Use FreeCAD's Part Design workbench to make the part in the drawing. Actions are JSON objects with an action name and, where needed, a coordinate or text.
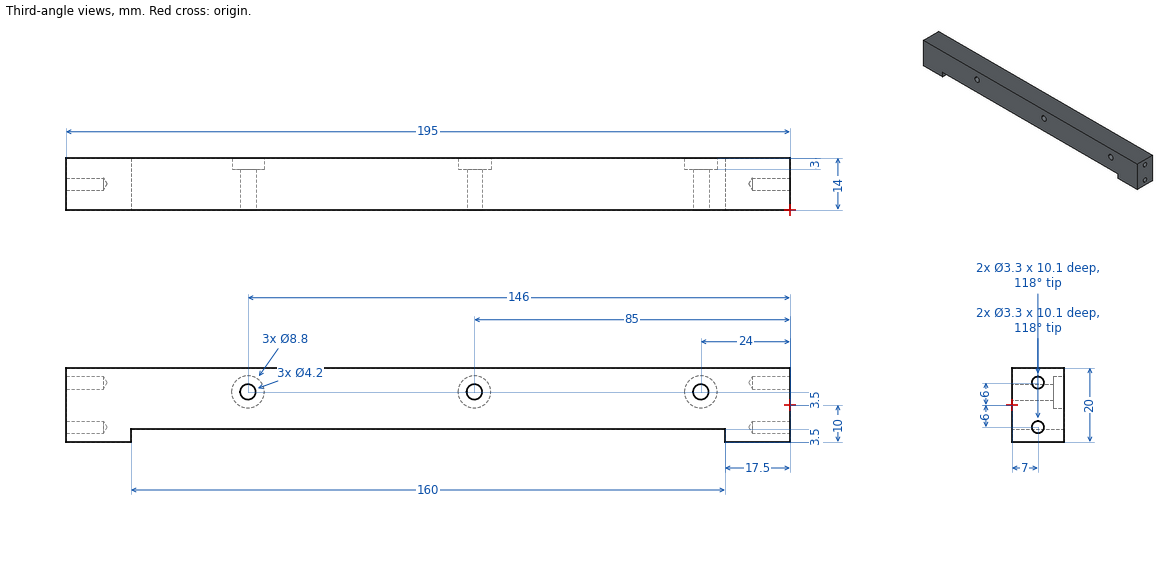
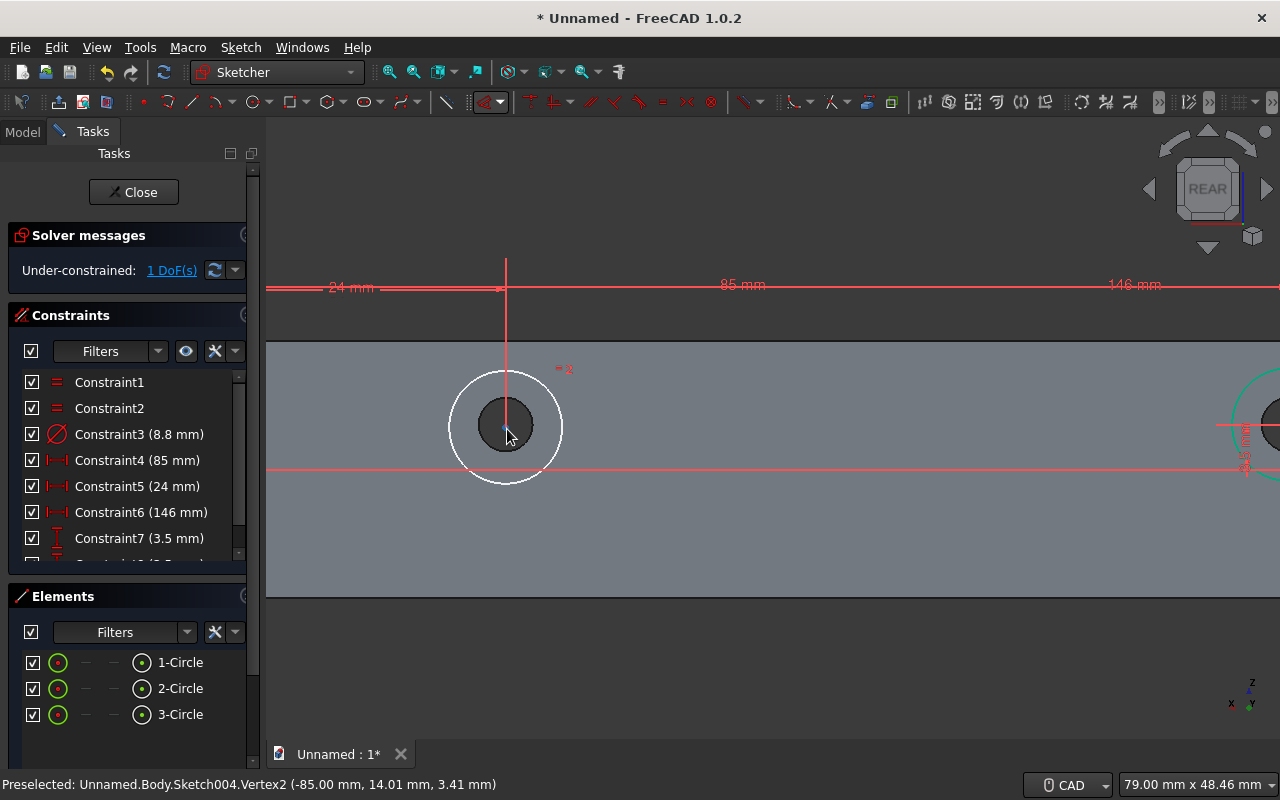
{"action": "left_click", "coordinate": [506, 427]}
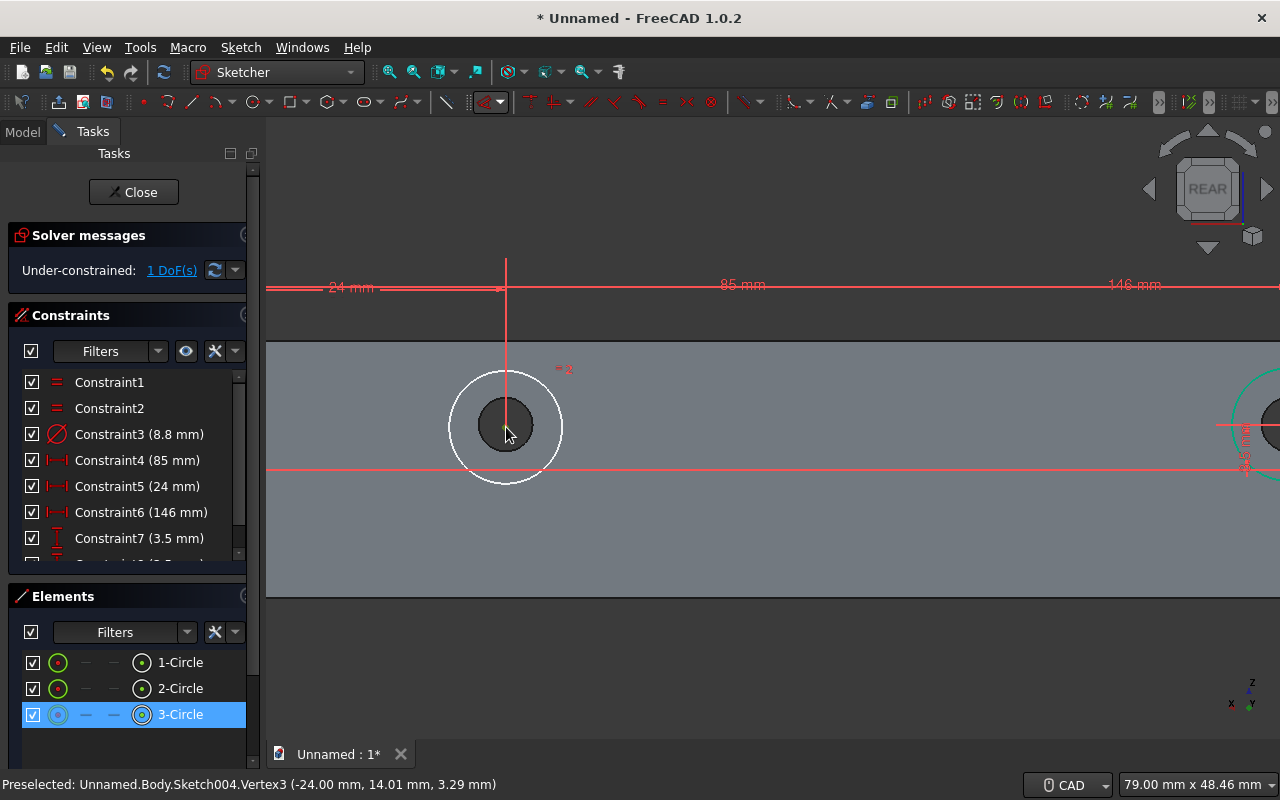
{"action": "key", "text": "i"}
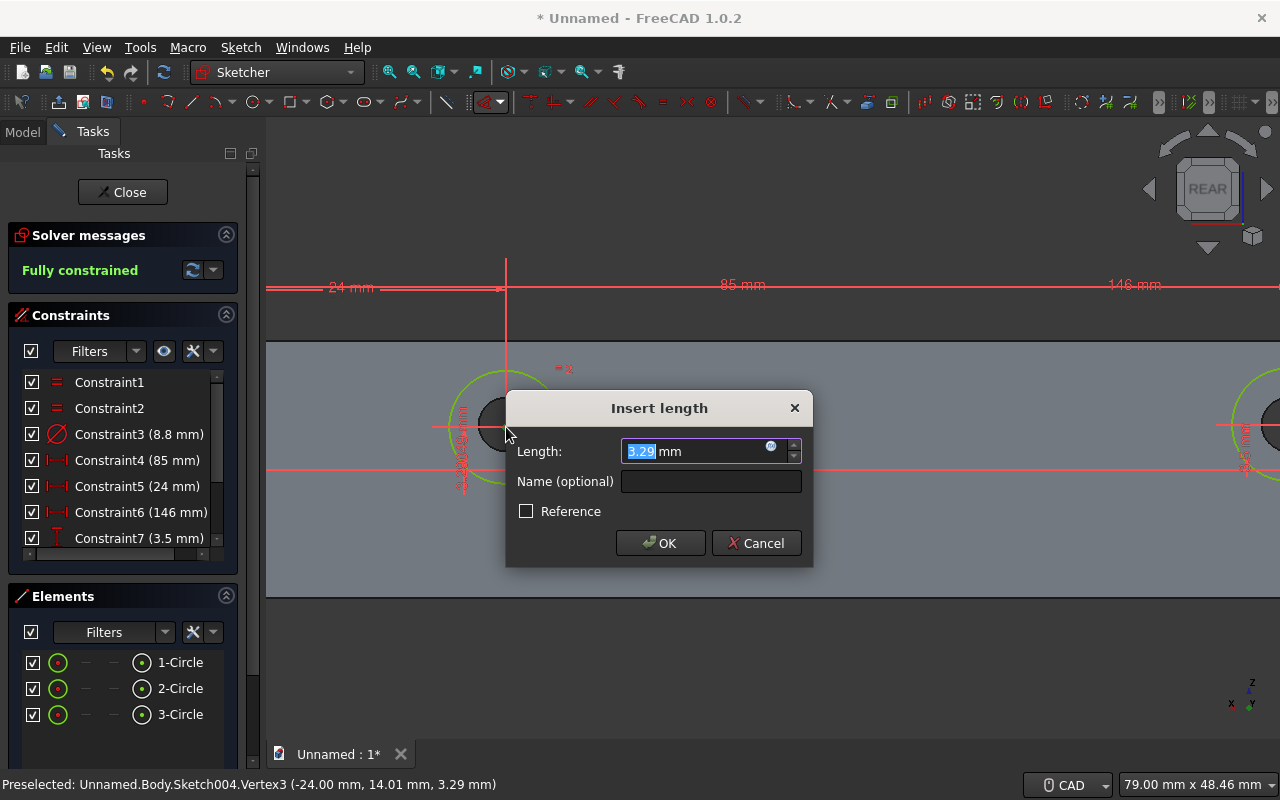
{"action": "type", "text": "3.5"}
{"action": "key", "text": "Return"}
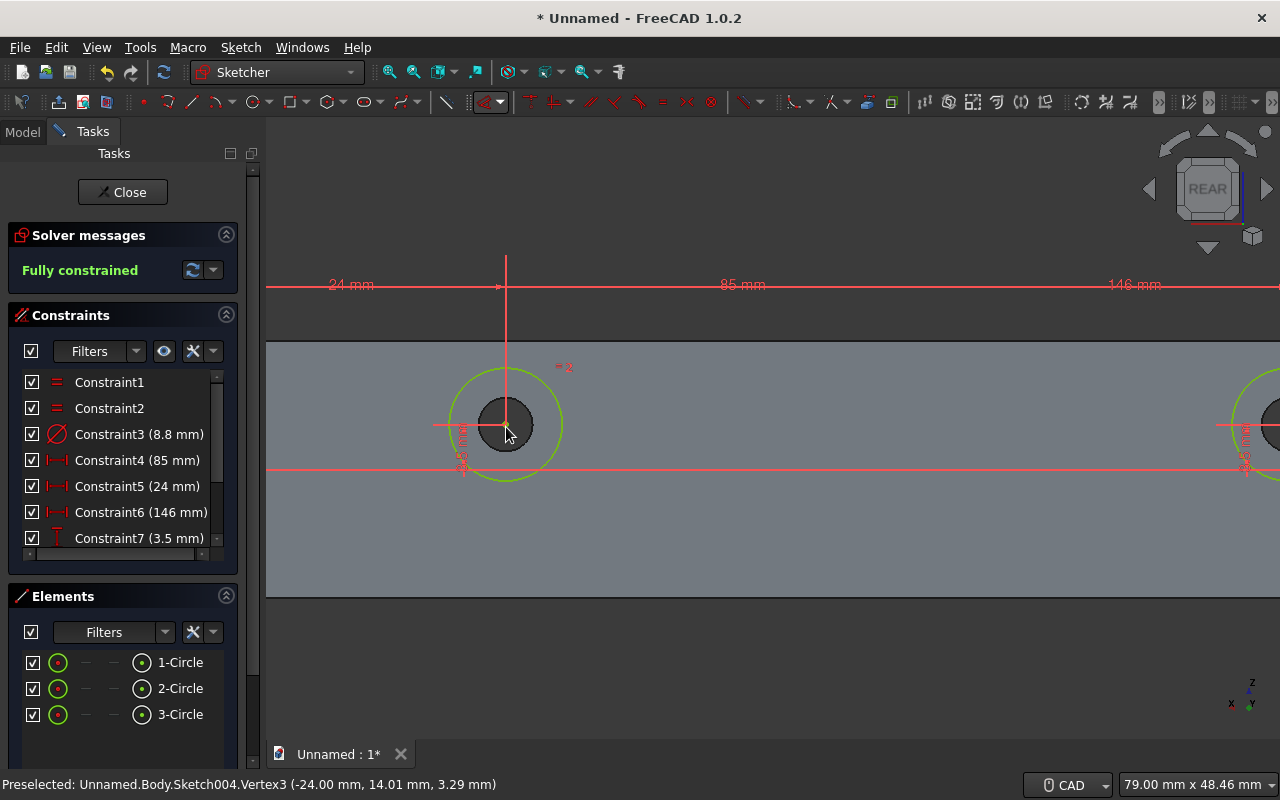
{"action": "left_click", "coordinate": [123, 192]}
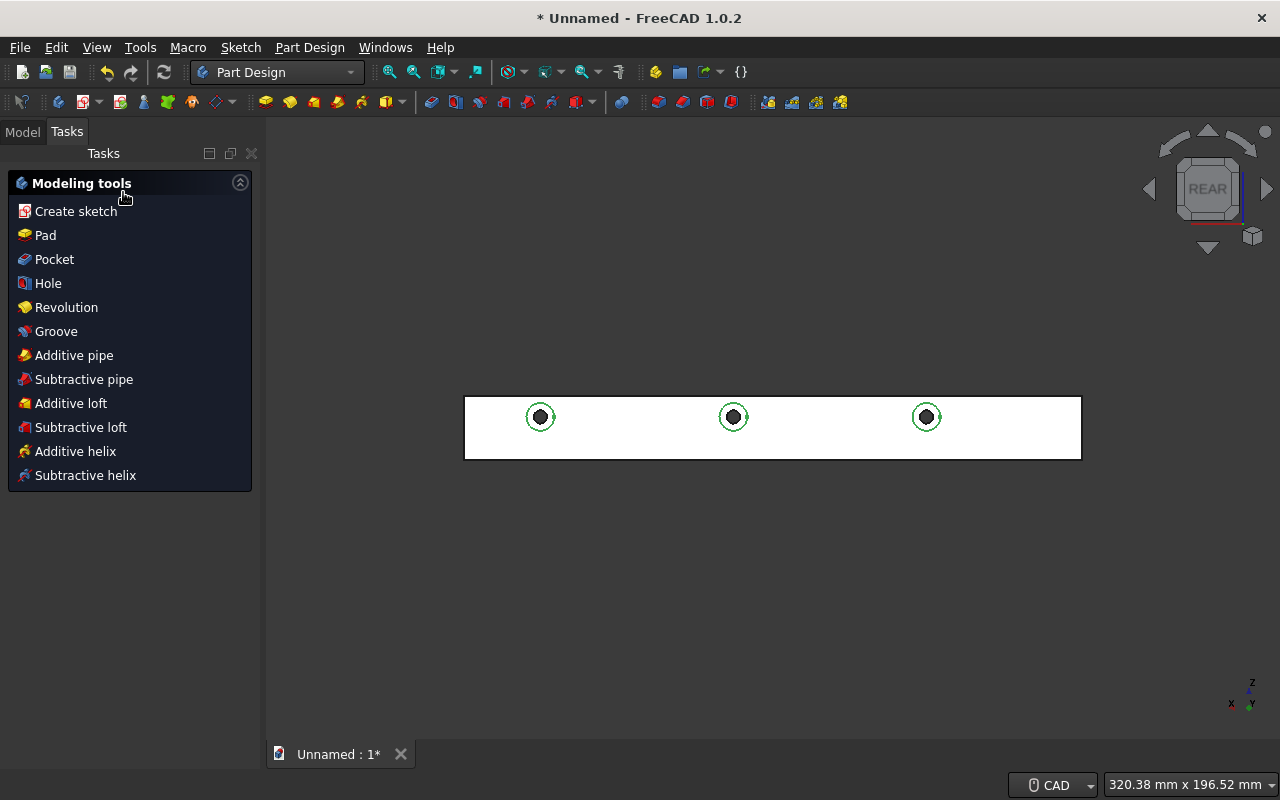
{"action": "left_click", "coordinate": [432, 102]}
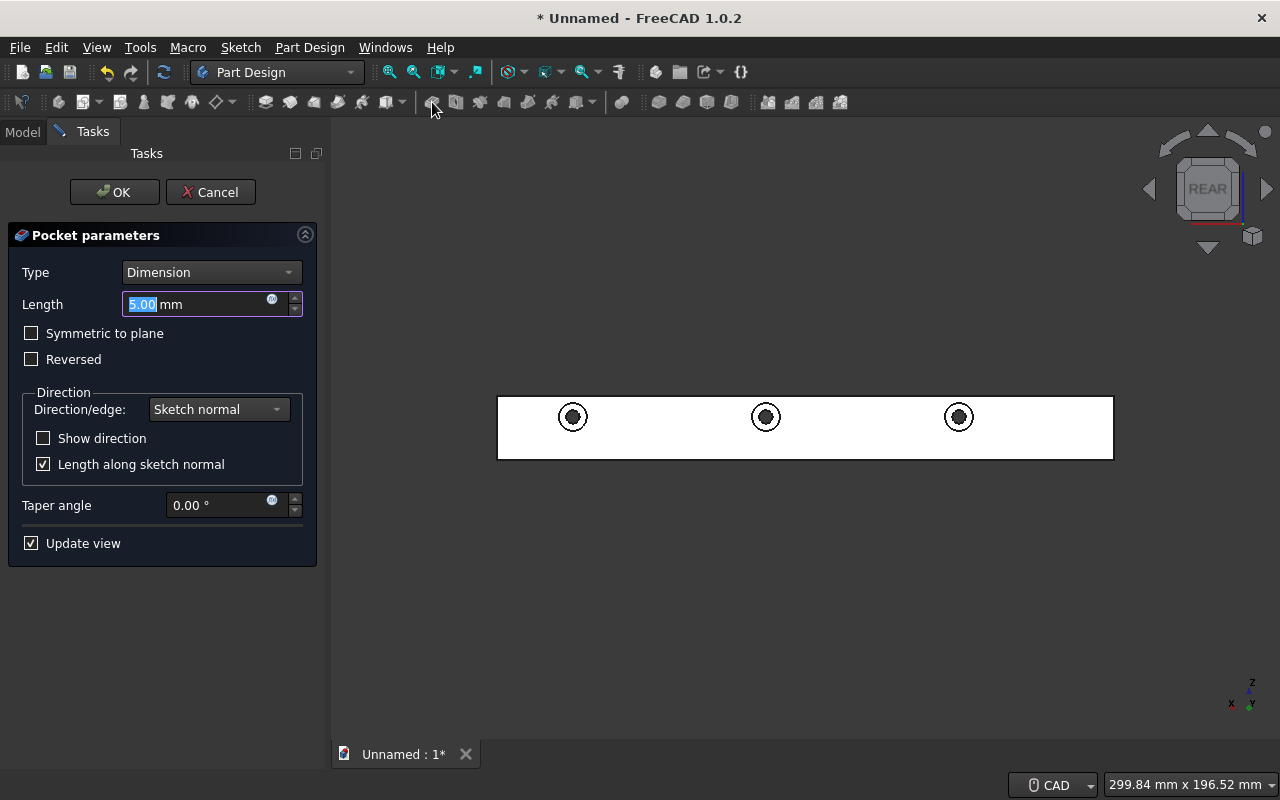
{"action": "type", "text": "3"}
{"action": "key", "text": "Tab"}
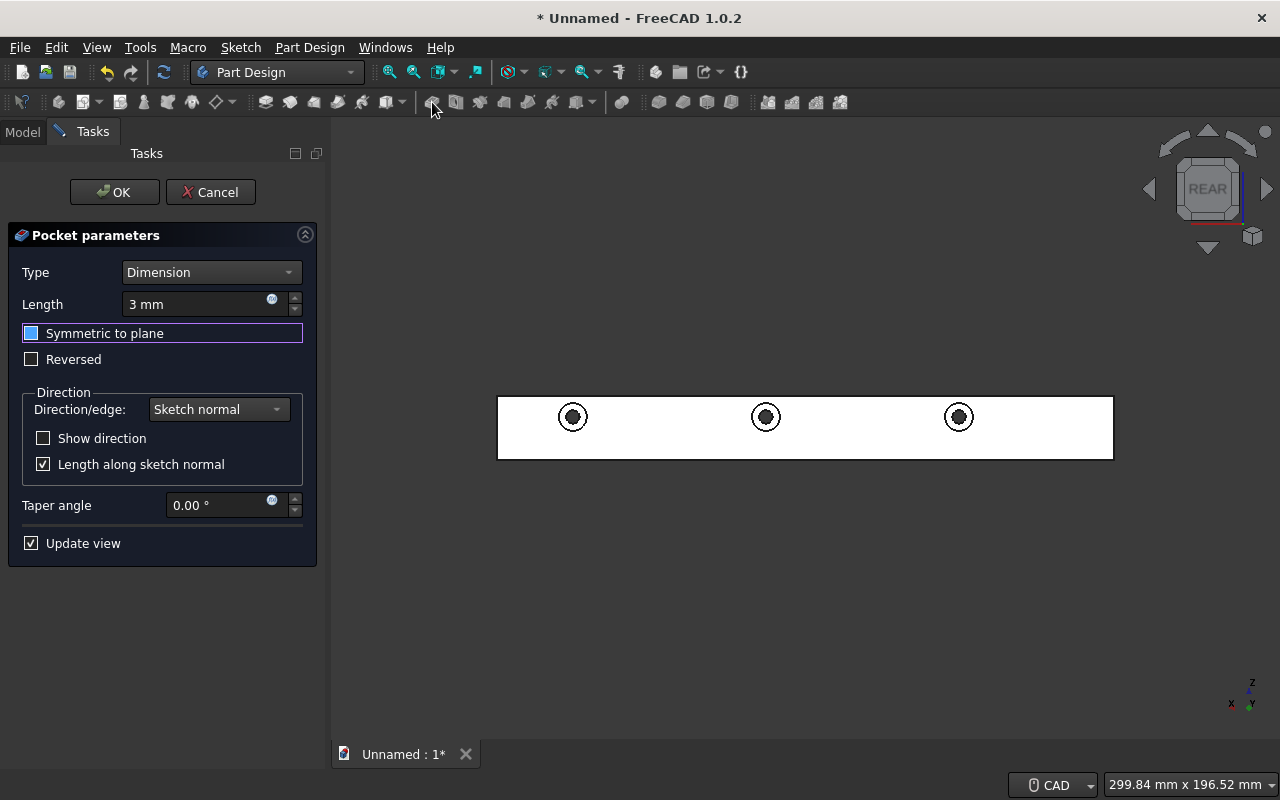
{"action": "left_click", "coordinate": [115, 192]}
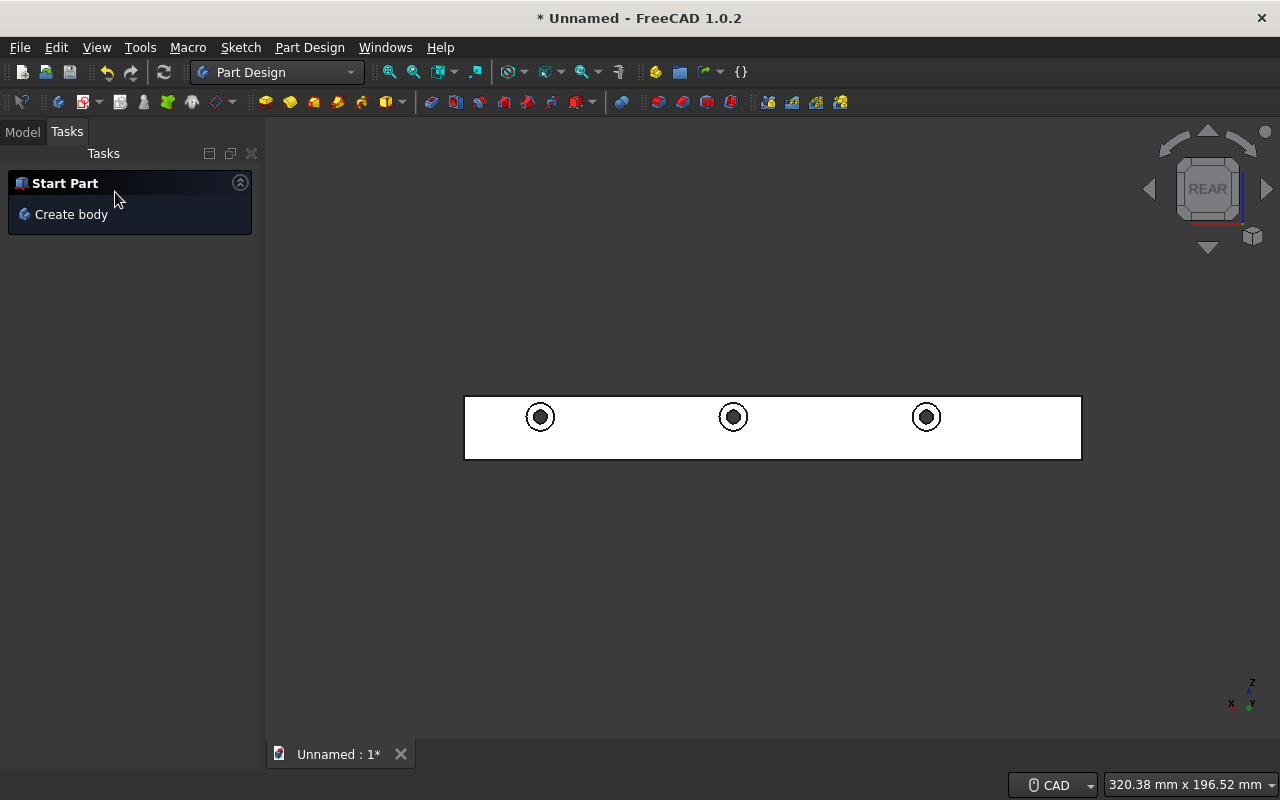
{"action": "left_click", "coordinate": [597, 427]}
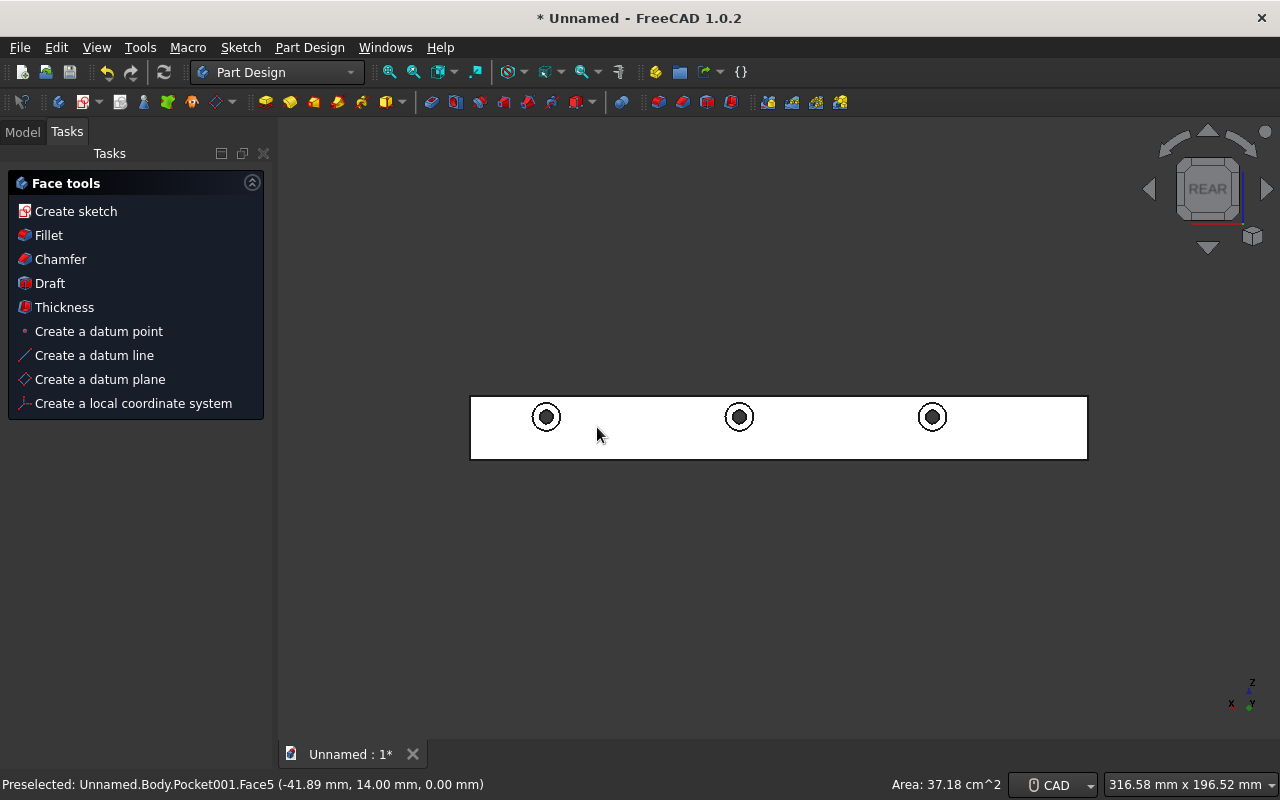
{"action": "left_click", "coordinate": [84, 102]}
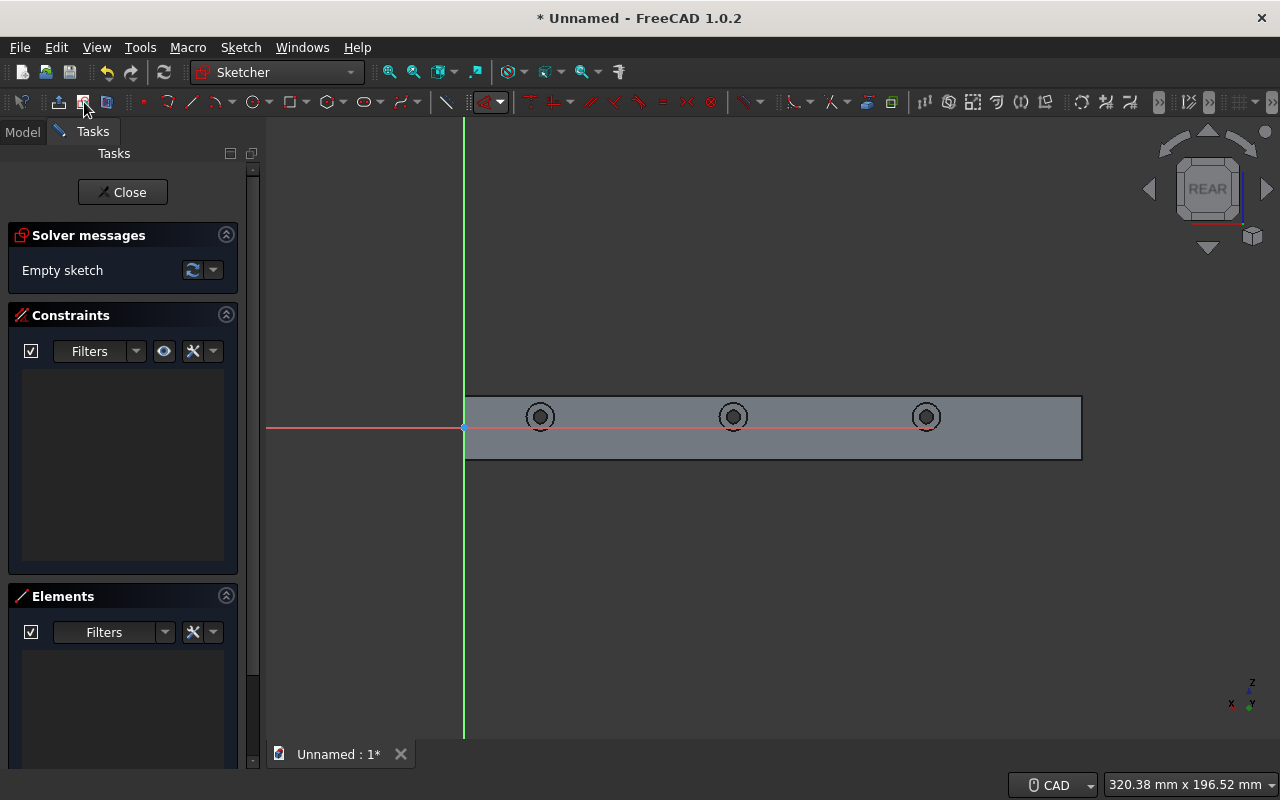
{"action": "key", "text": "g r"}